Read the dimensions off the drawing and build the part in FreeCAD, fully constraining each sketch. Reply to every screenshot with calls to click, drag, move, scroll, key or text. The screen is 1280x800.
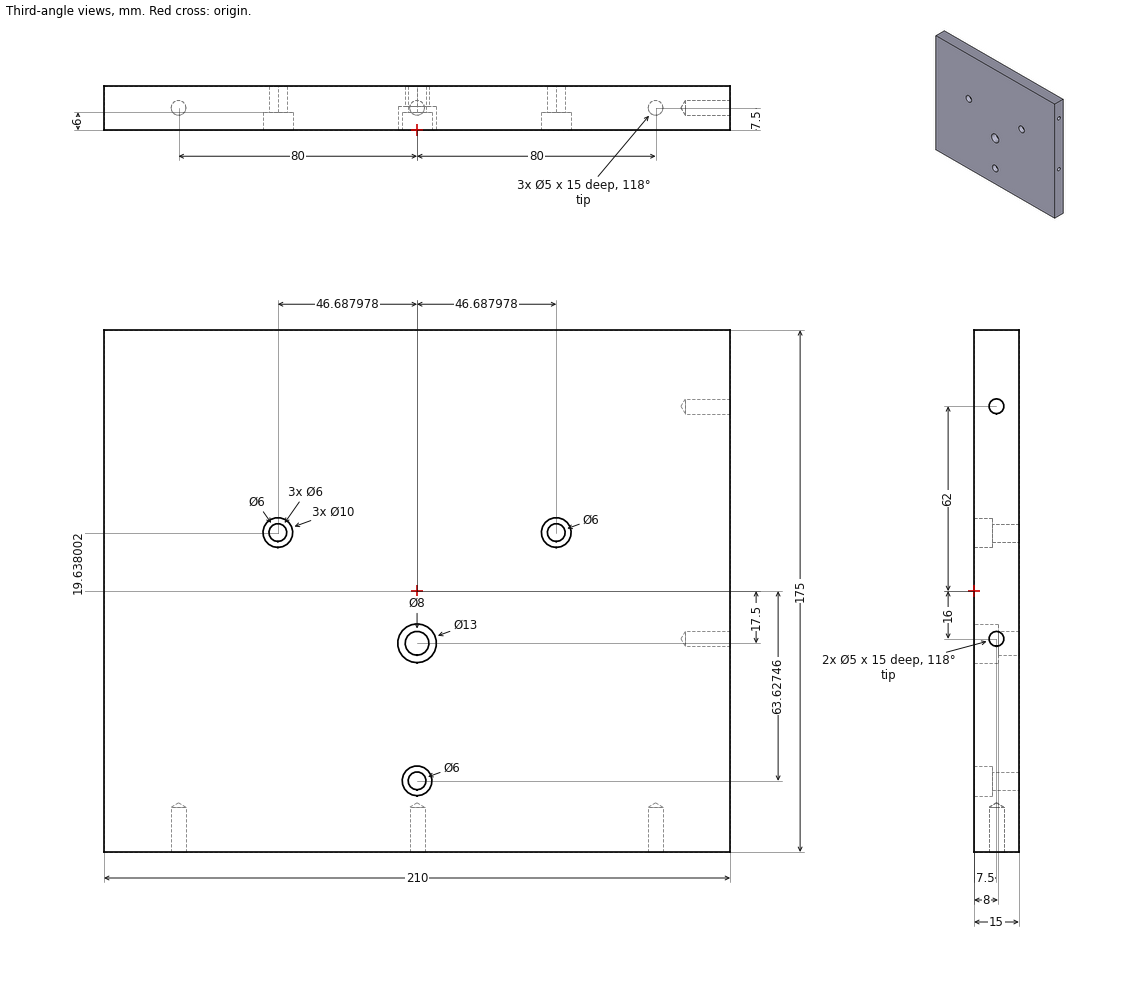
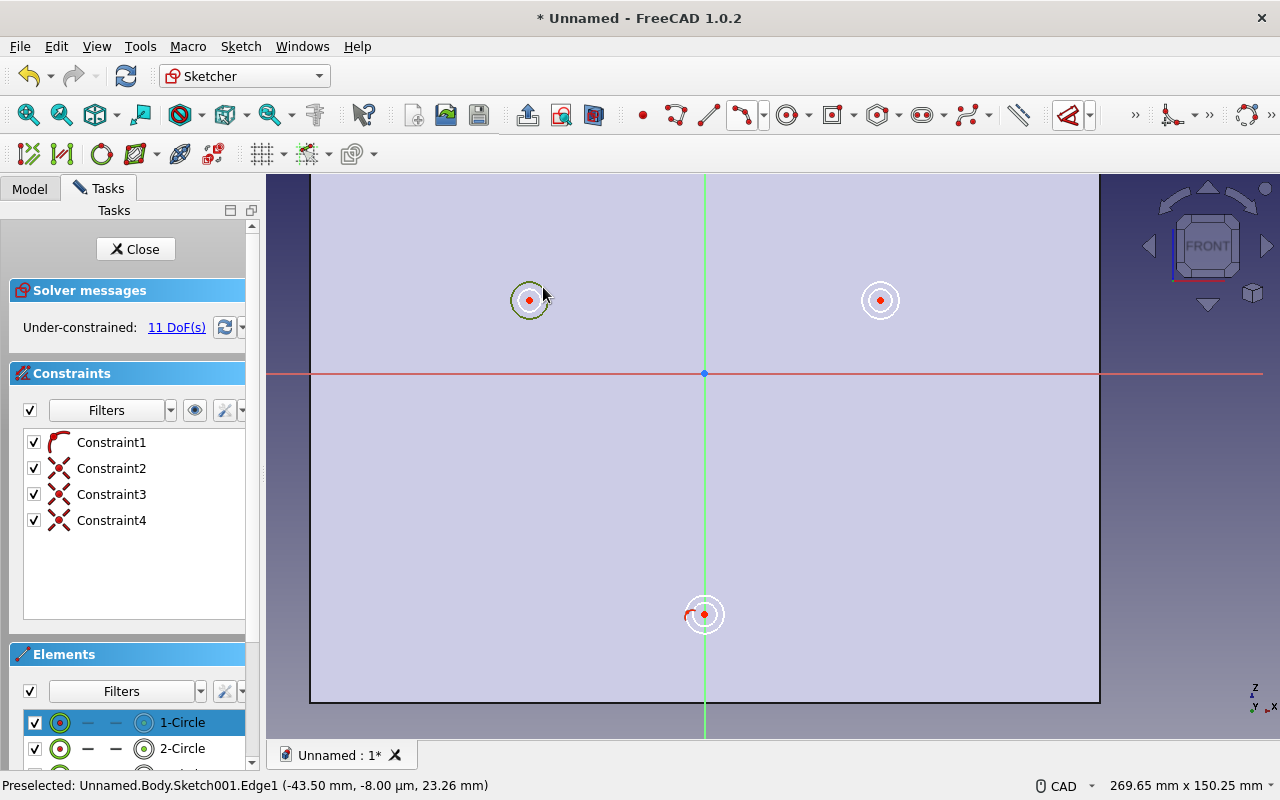
scroll(894, 288, up, 4)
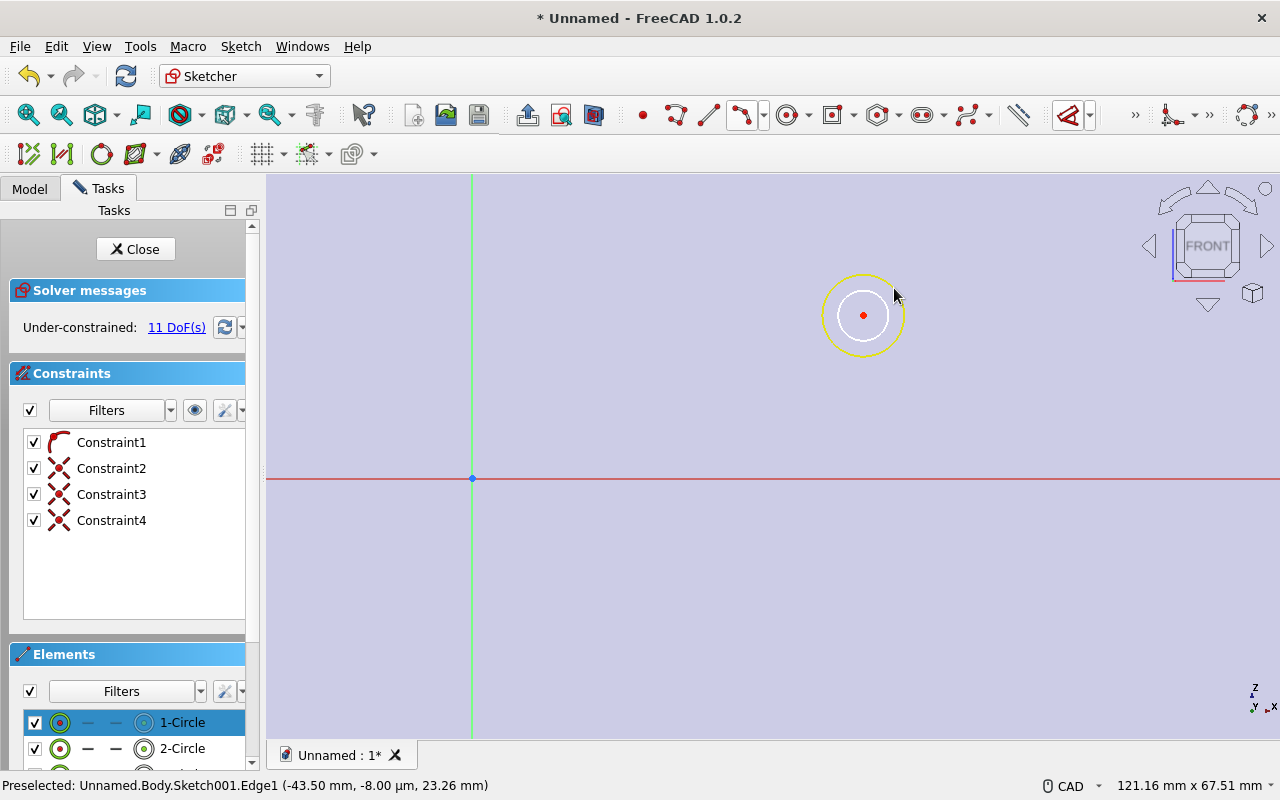
click(892, 287)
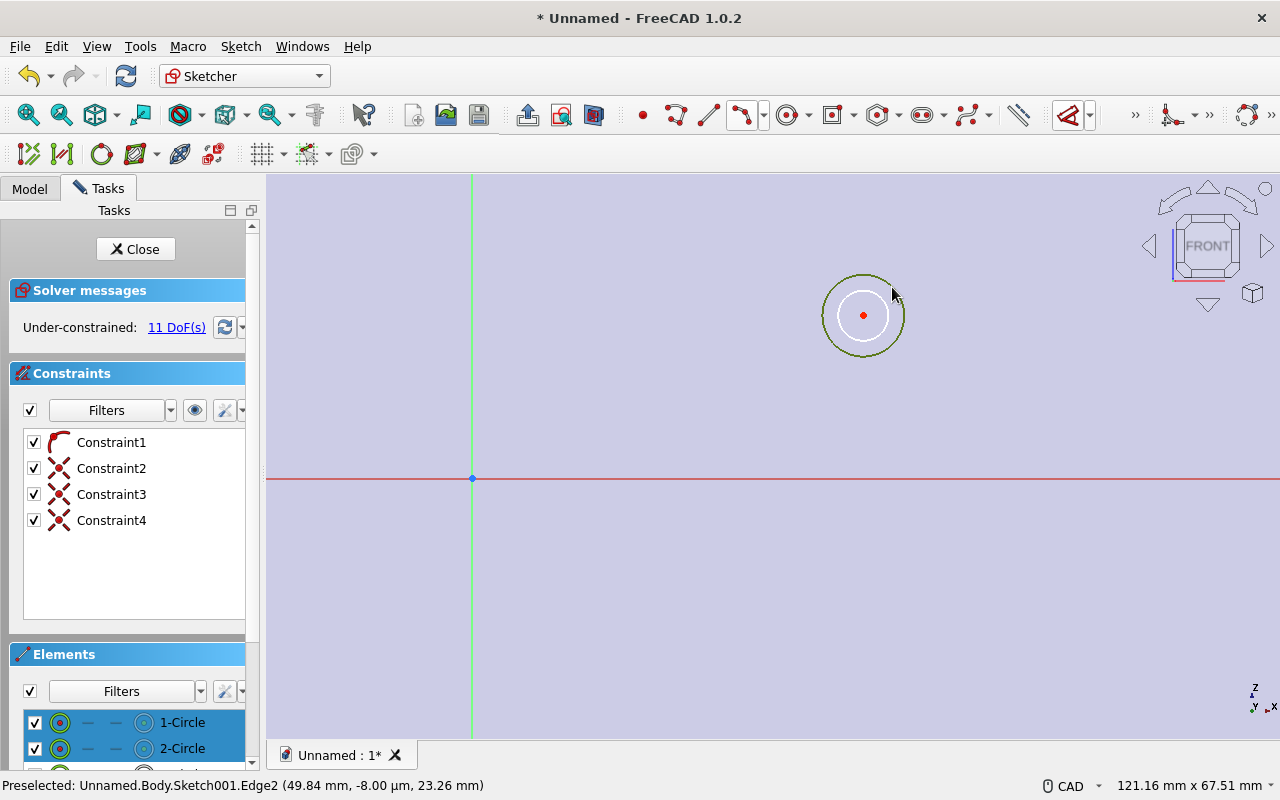
scroll(894, 288, down, 4)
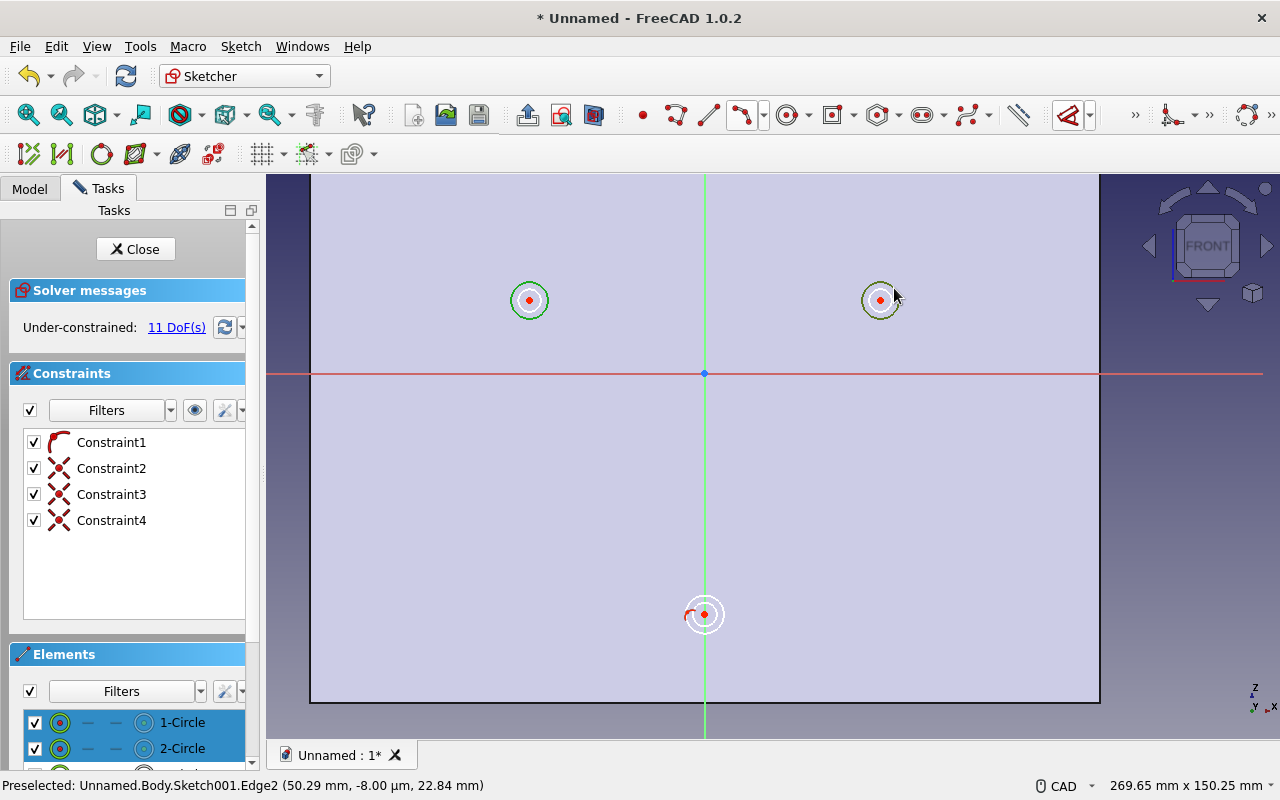
scroll(718, 601, up, 4)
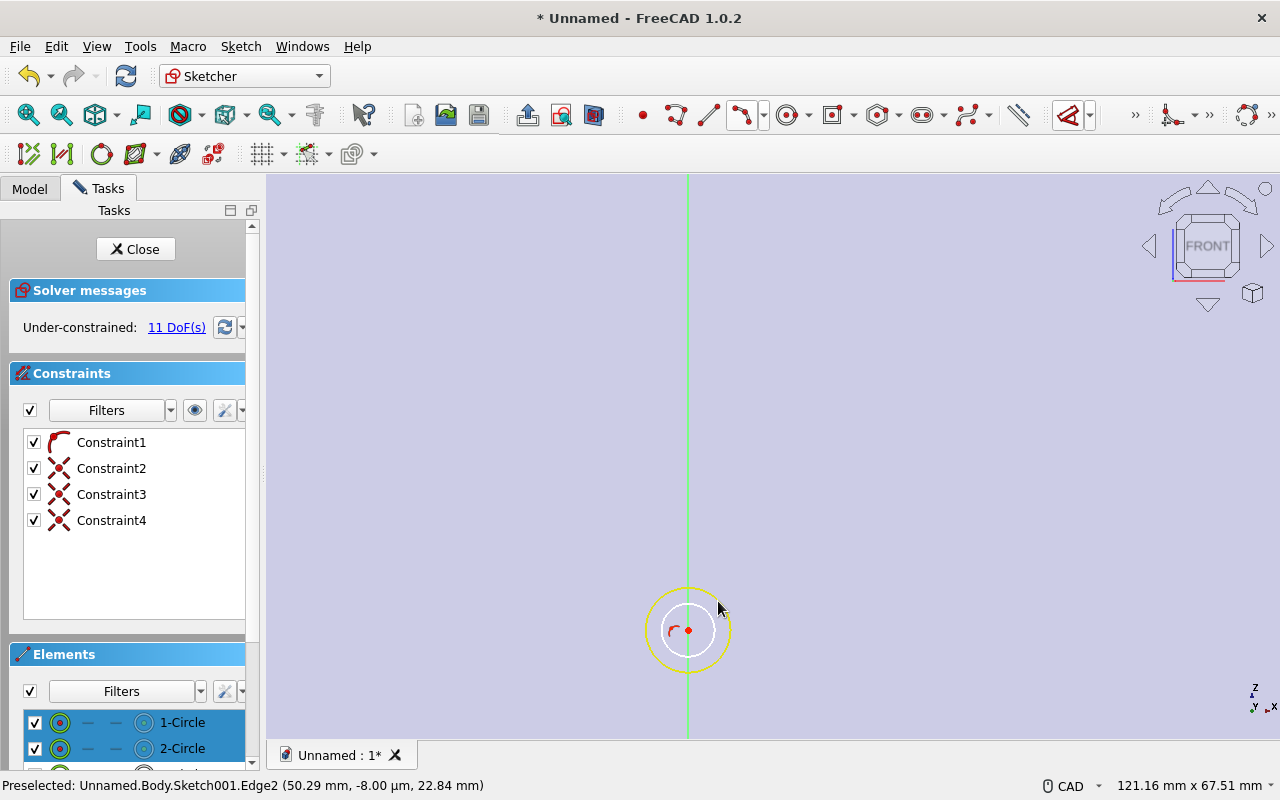
click(718, 600)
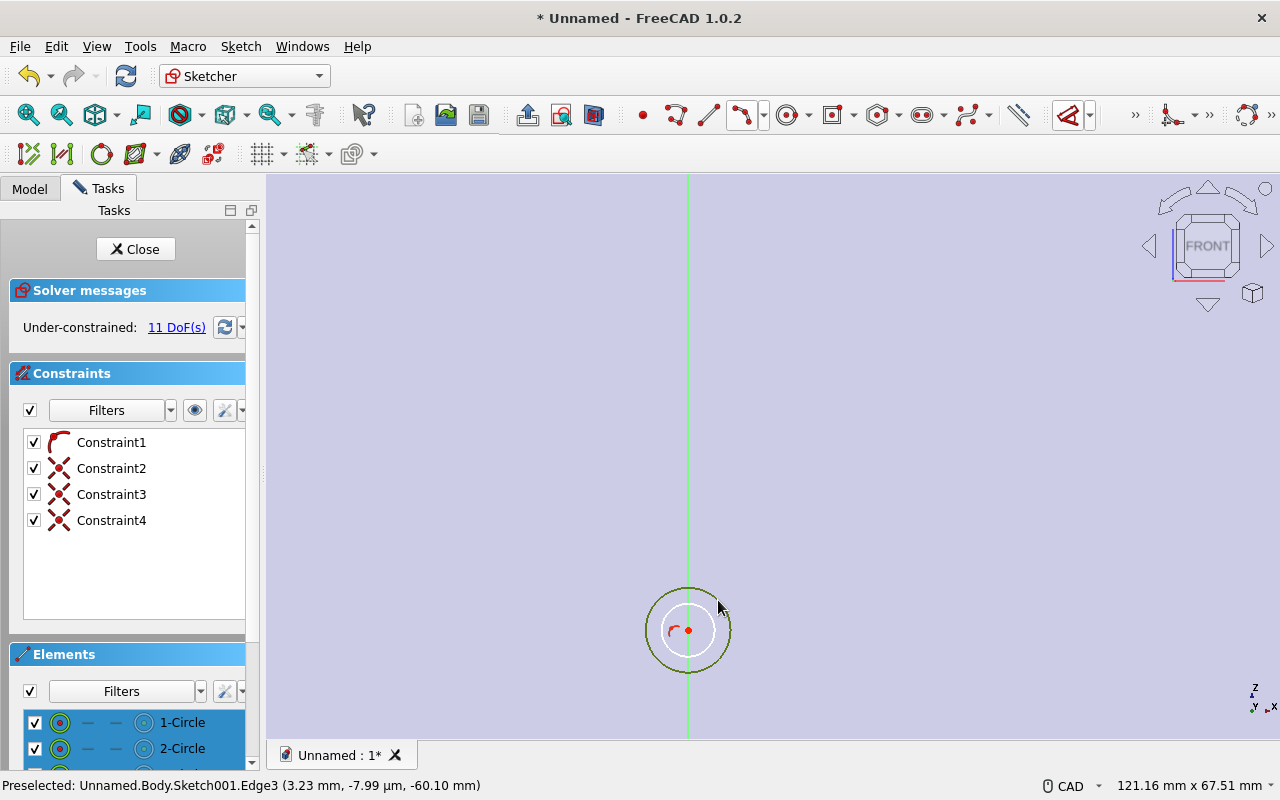
key(e)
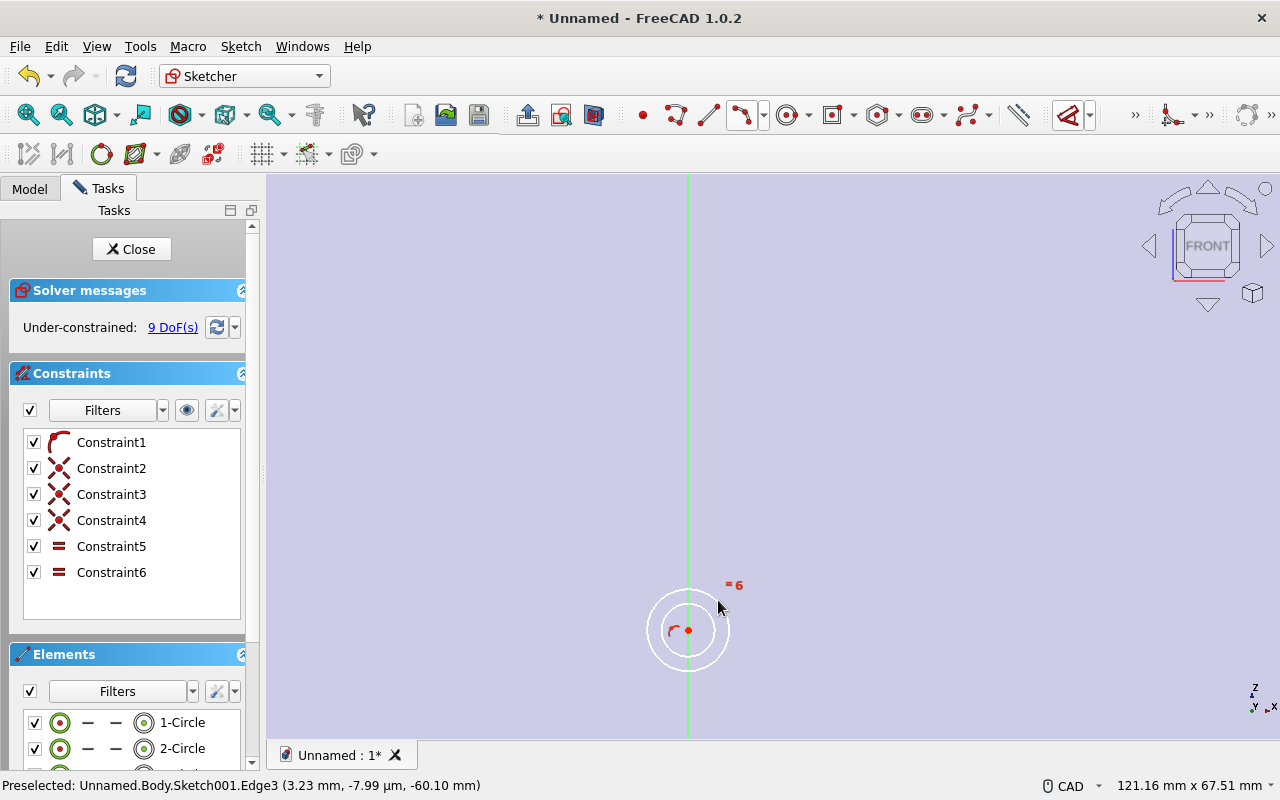
scroll(718, 602, down, 4)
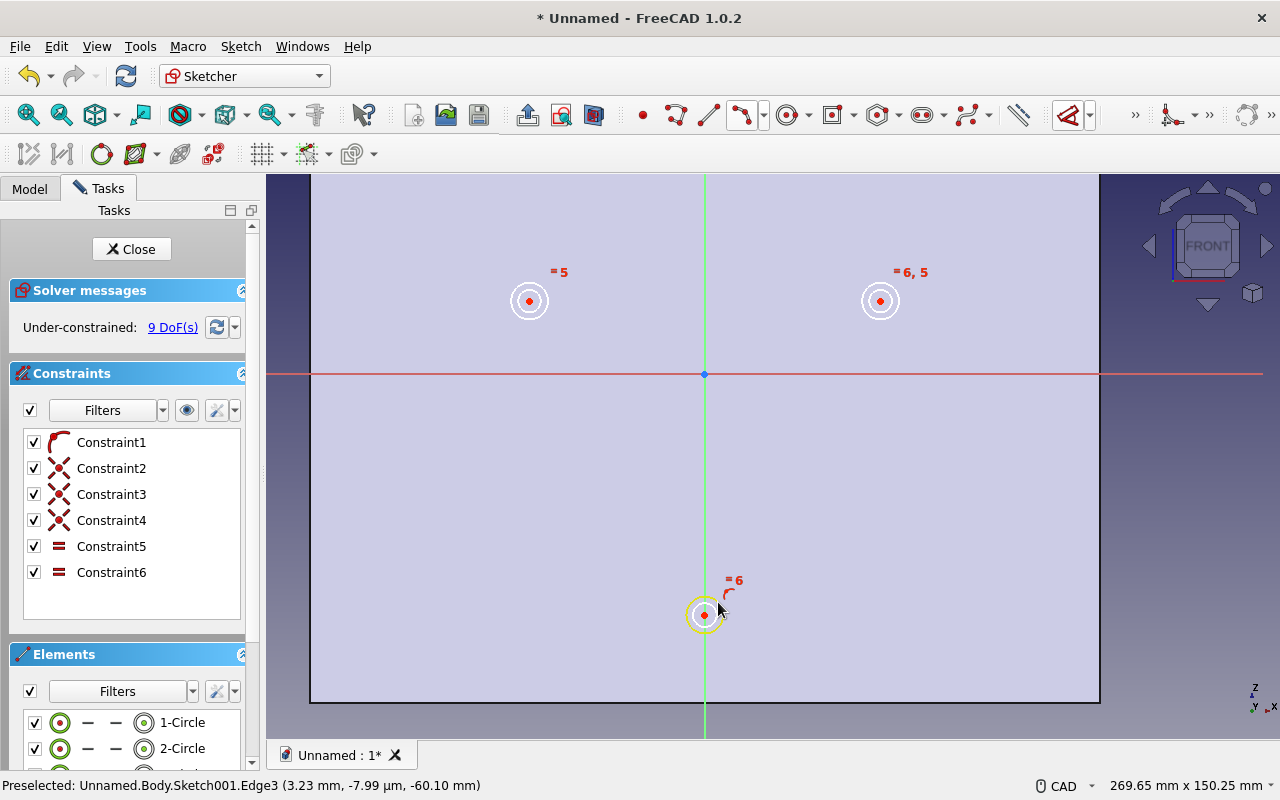
scroll(537, 293, up, 4)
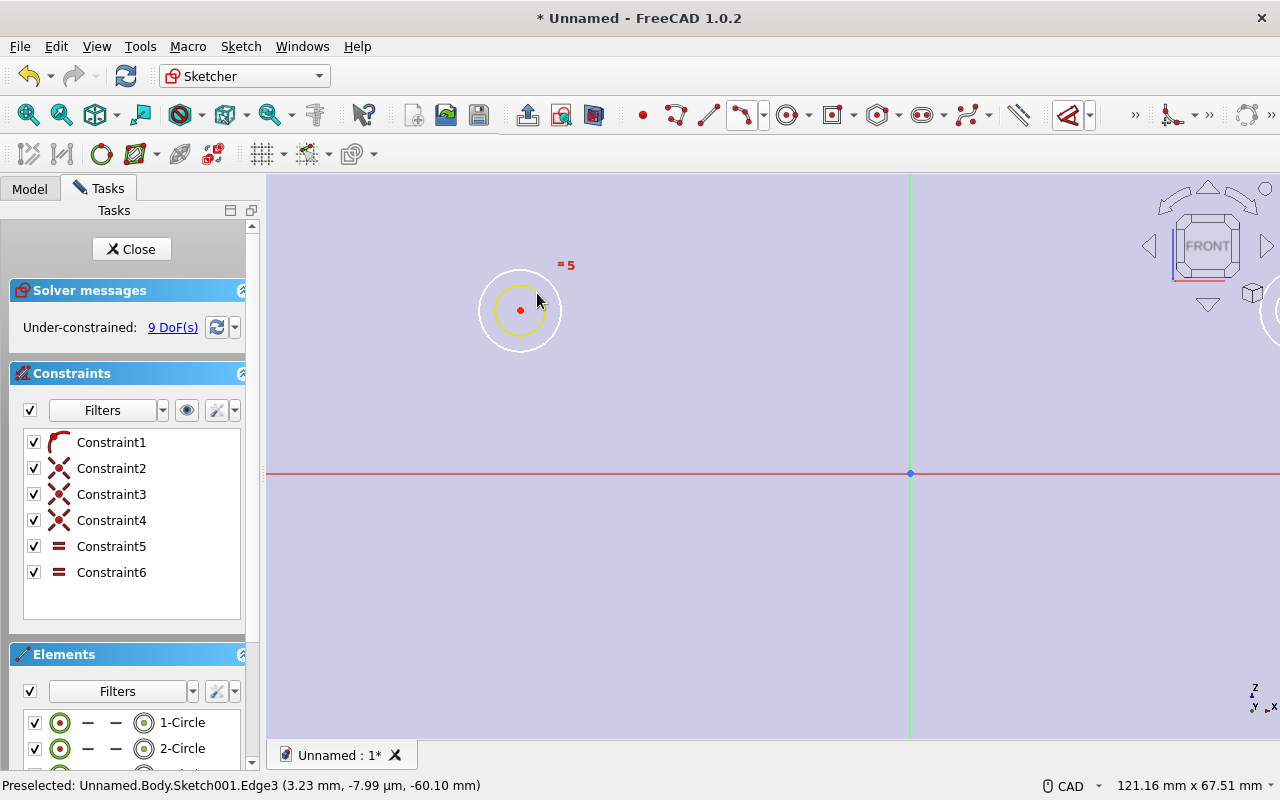
click(538, 293)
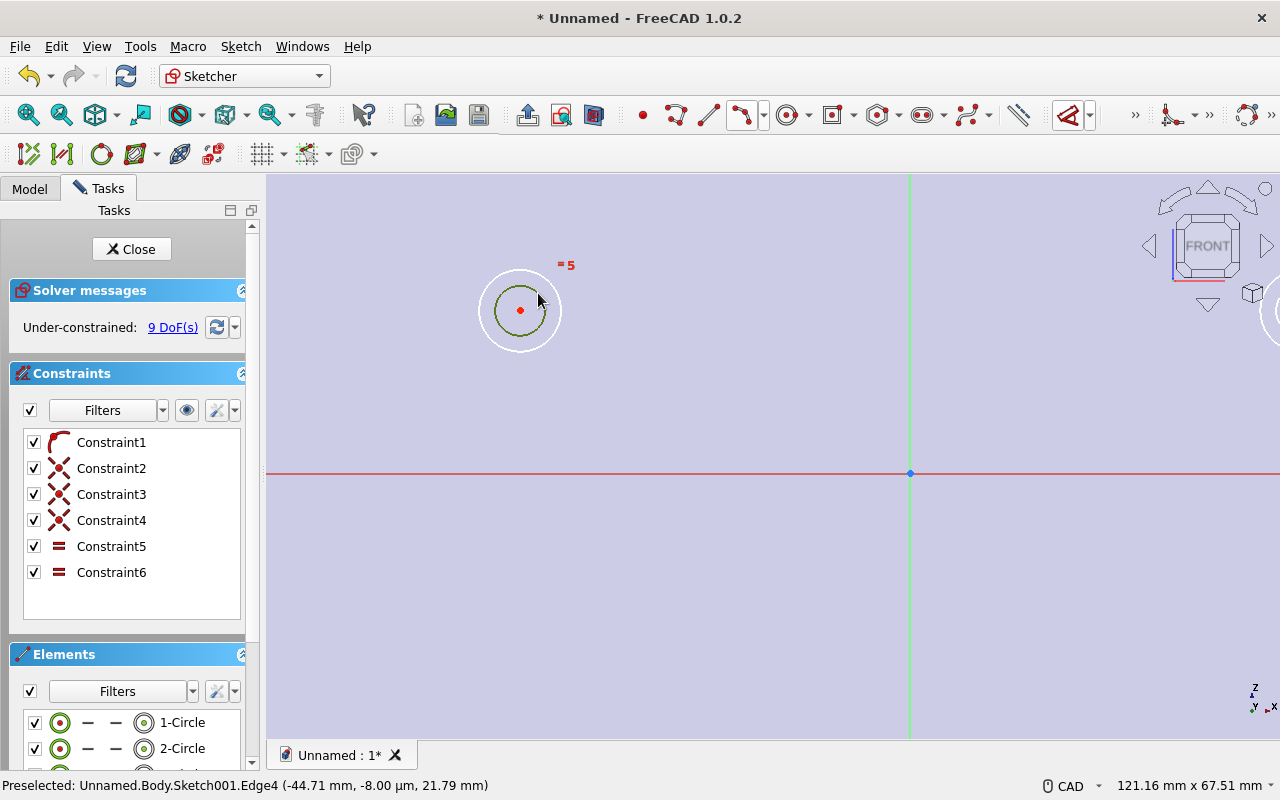
scroll(537, 292, down, 4)